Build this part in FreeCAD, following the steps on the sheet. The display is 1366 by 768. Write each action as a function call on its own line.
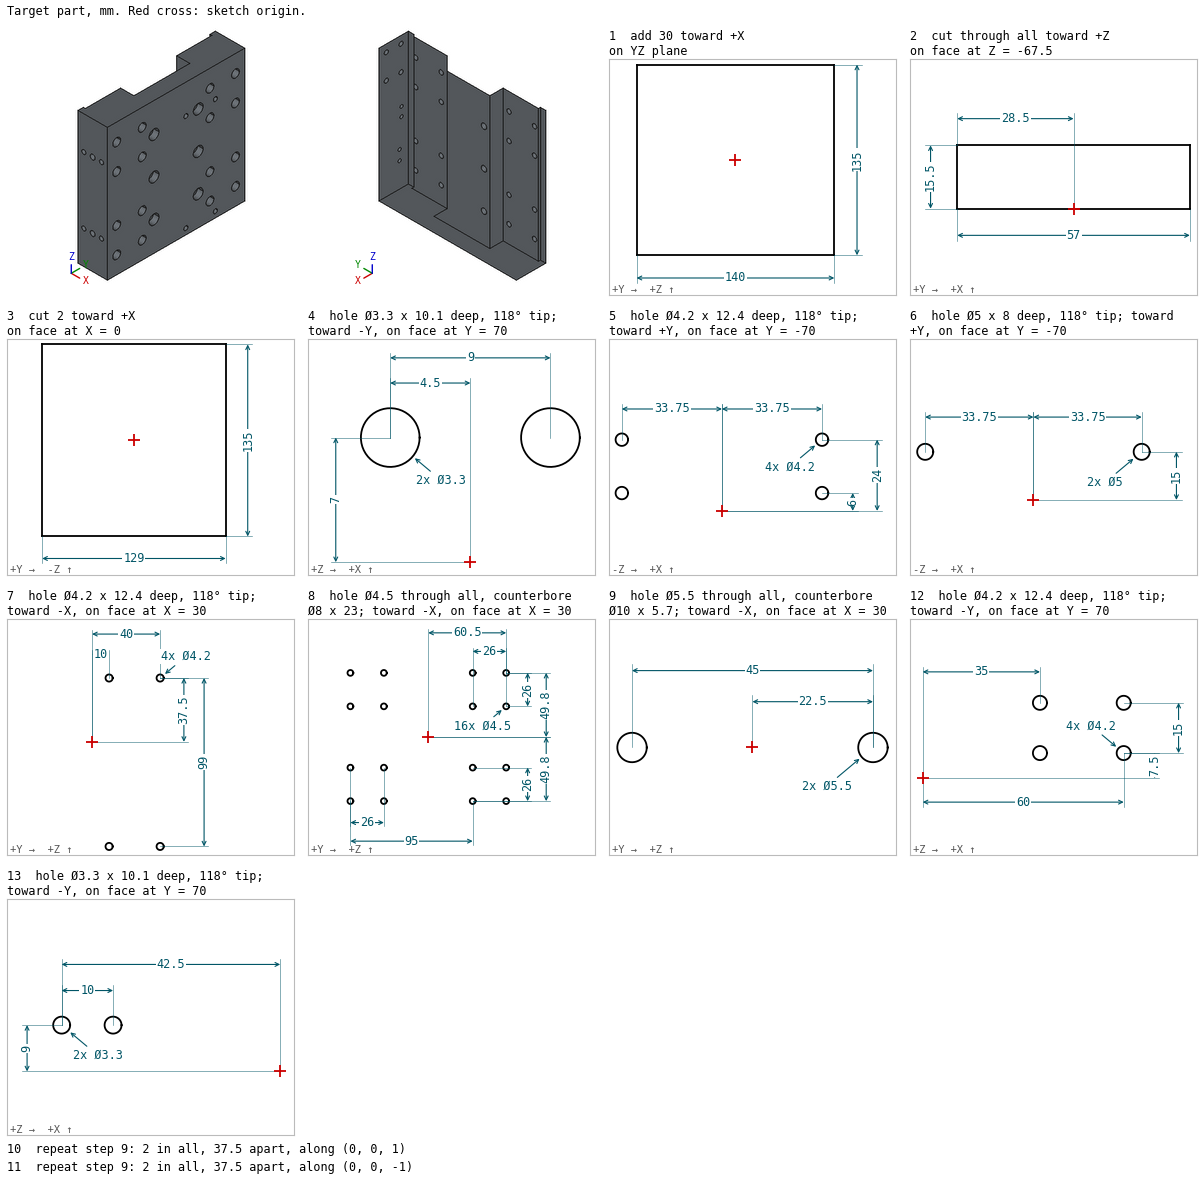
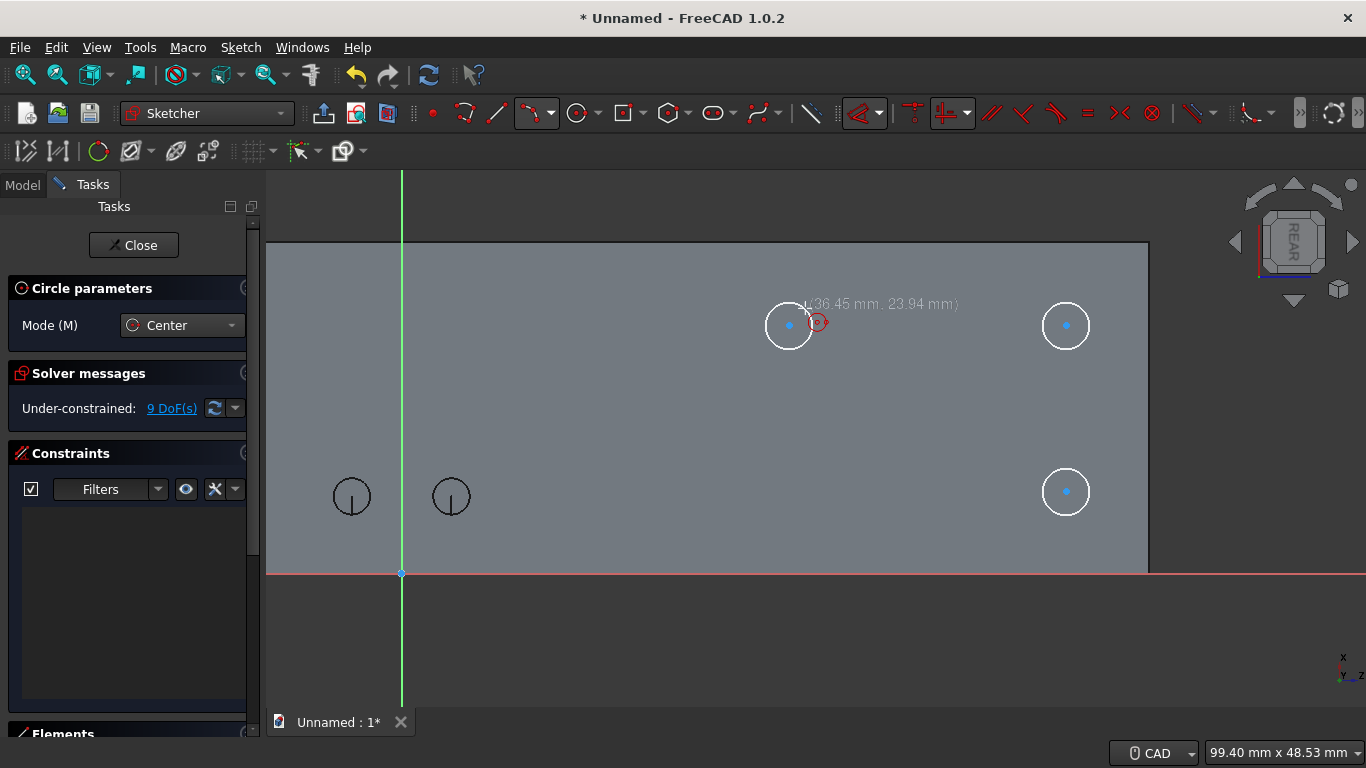
click(789, 491)
click(805, 474)
key(Escape)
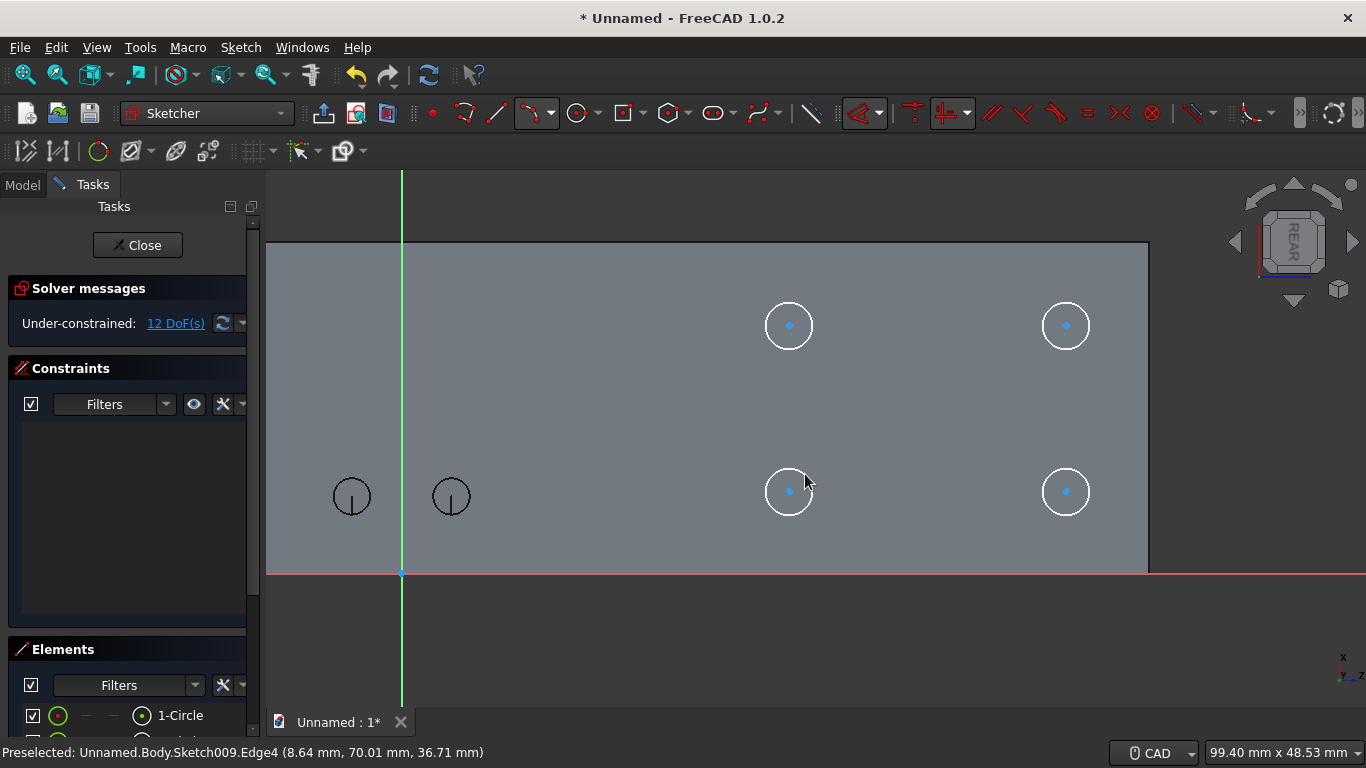
click(1082, 475)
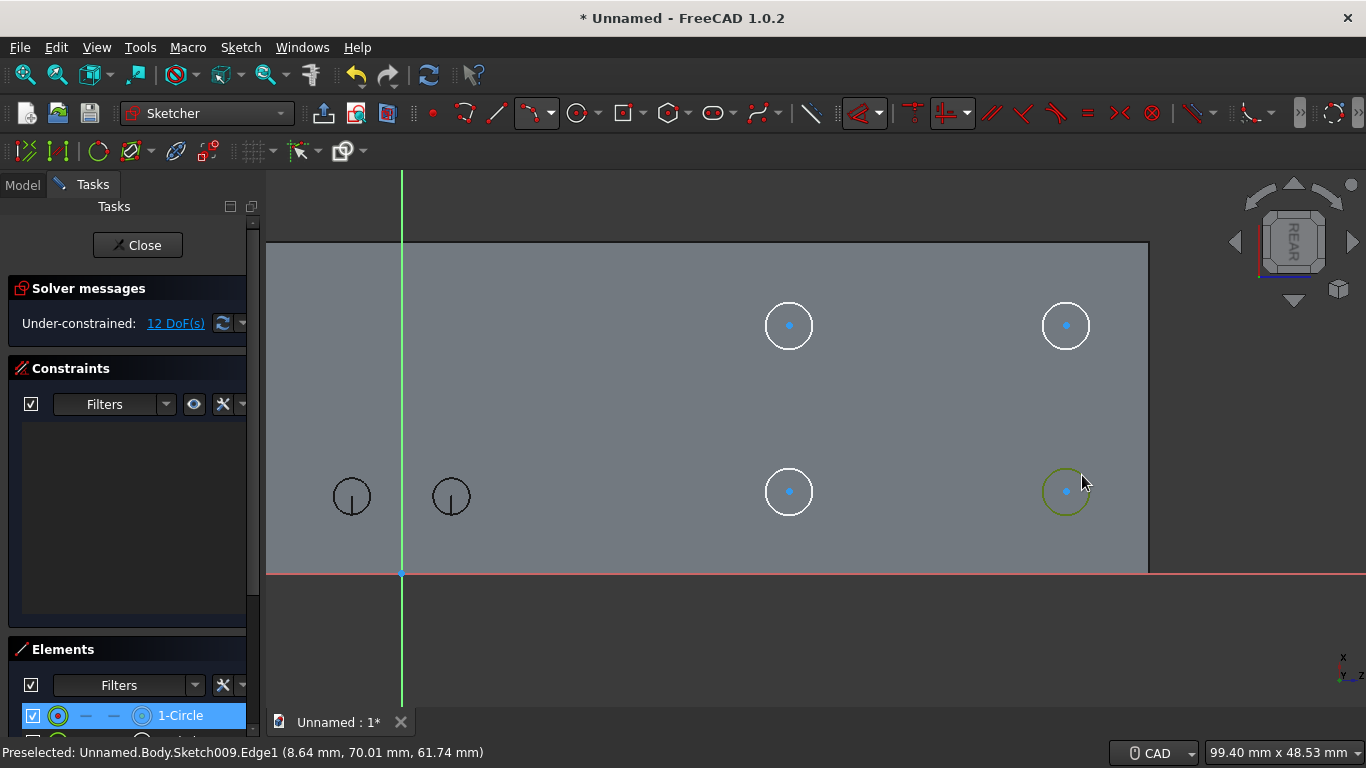
click(1082, 309)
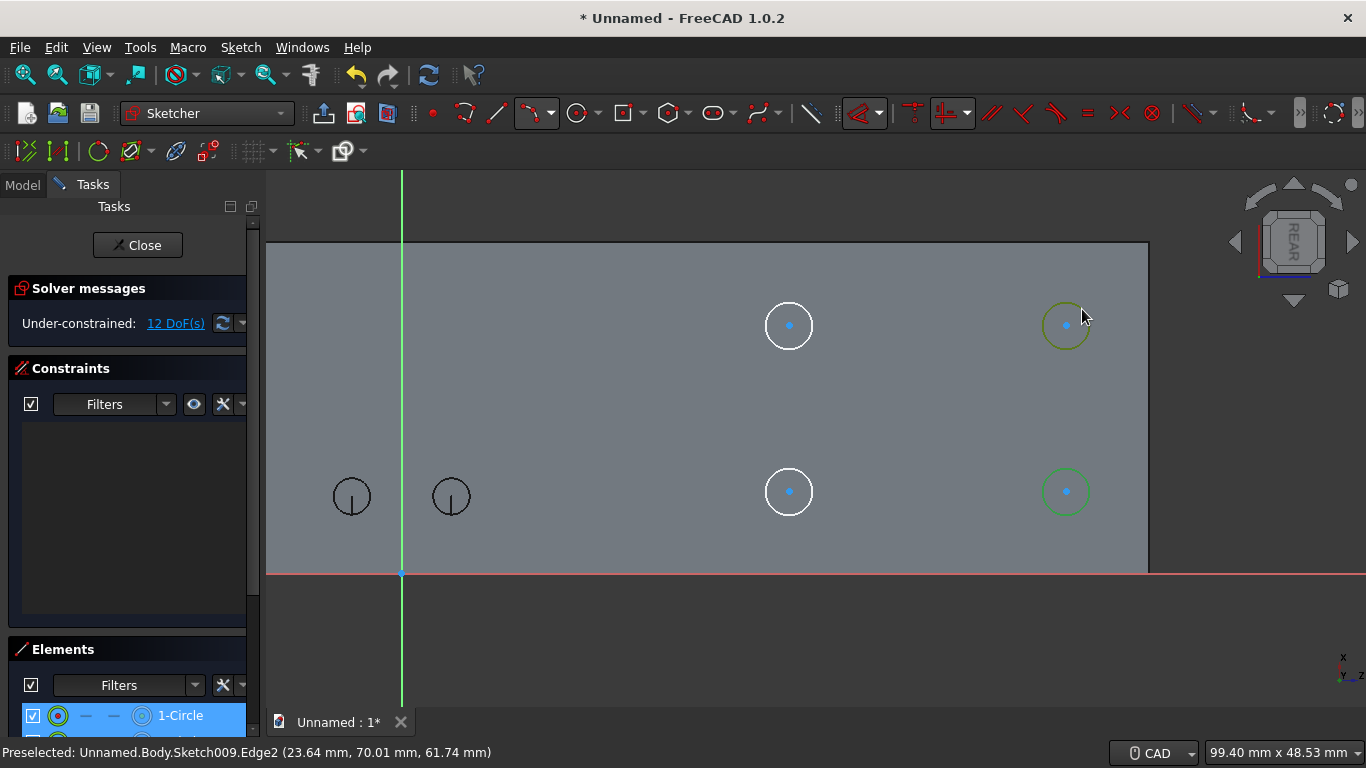
click(805, 309)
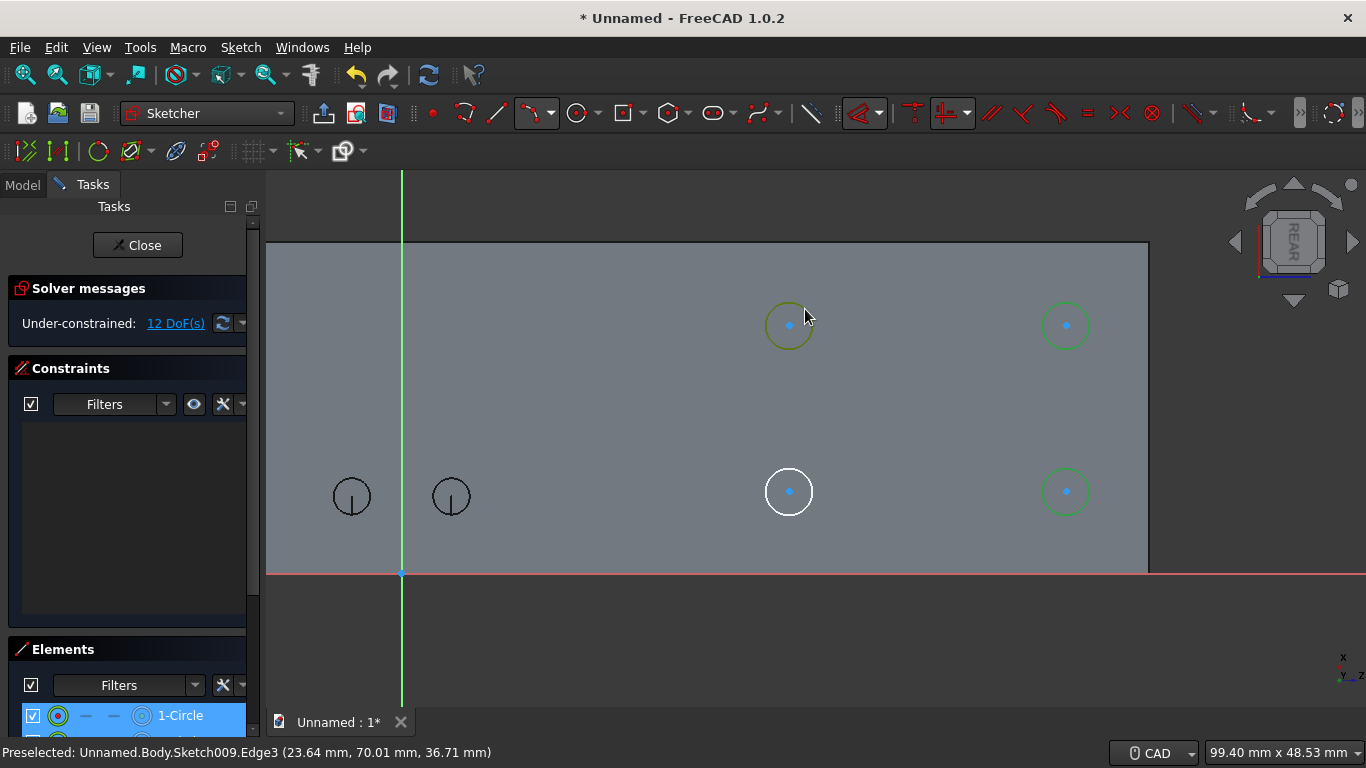
click(805, 475)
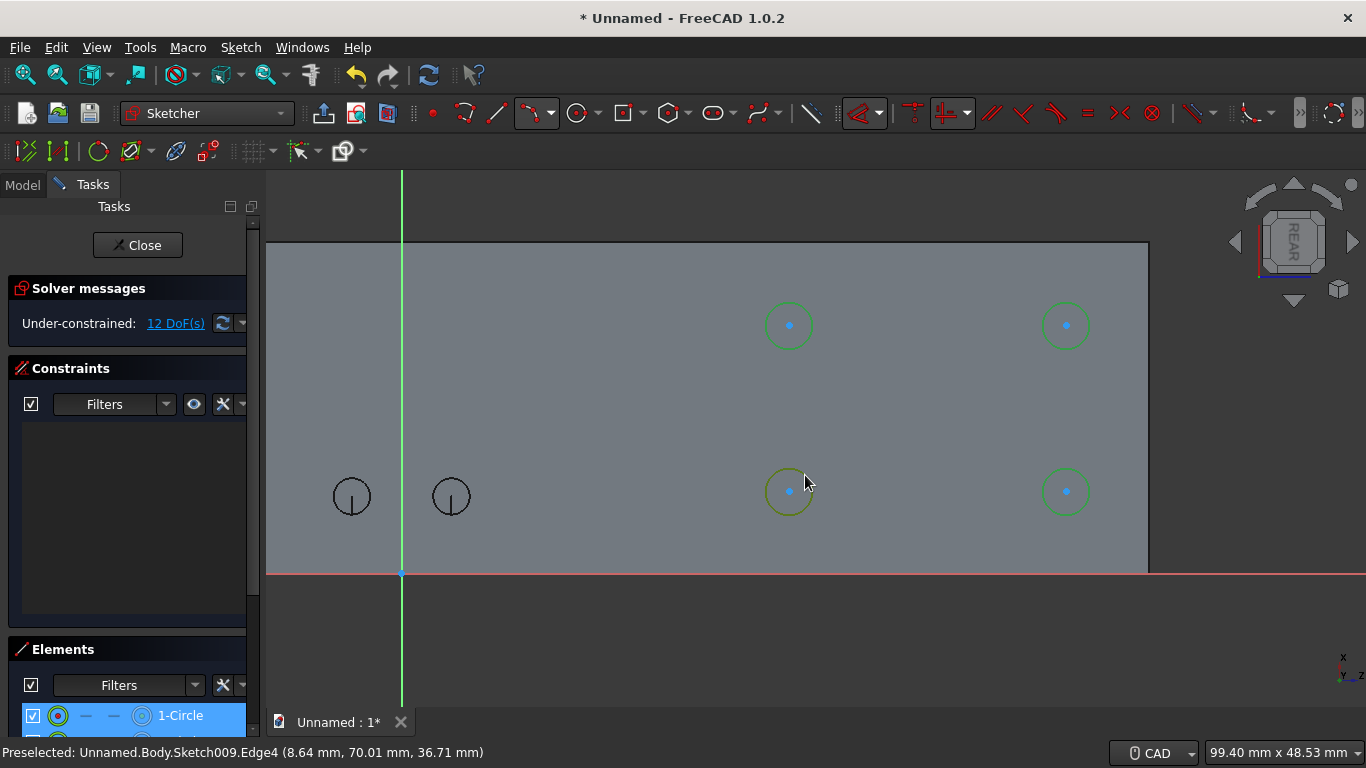
click(1088, 114)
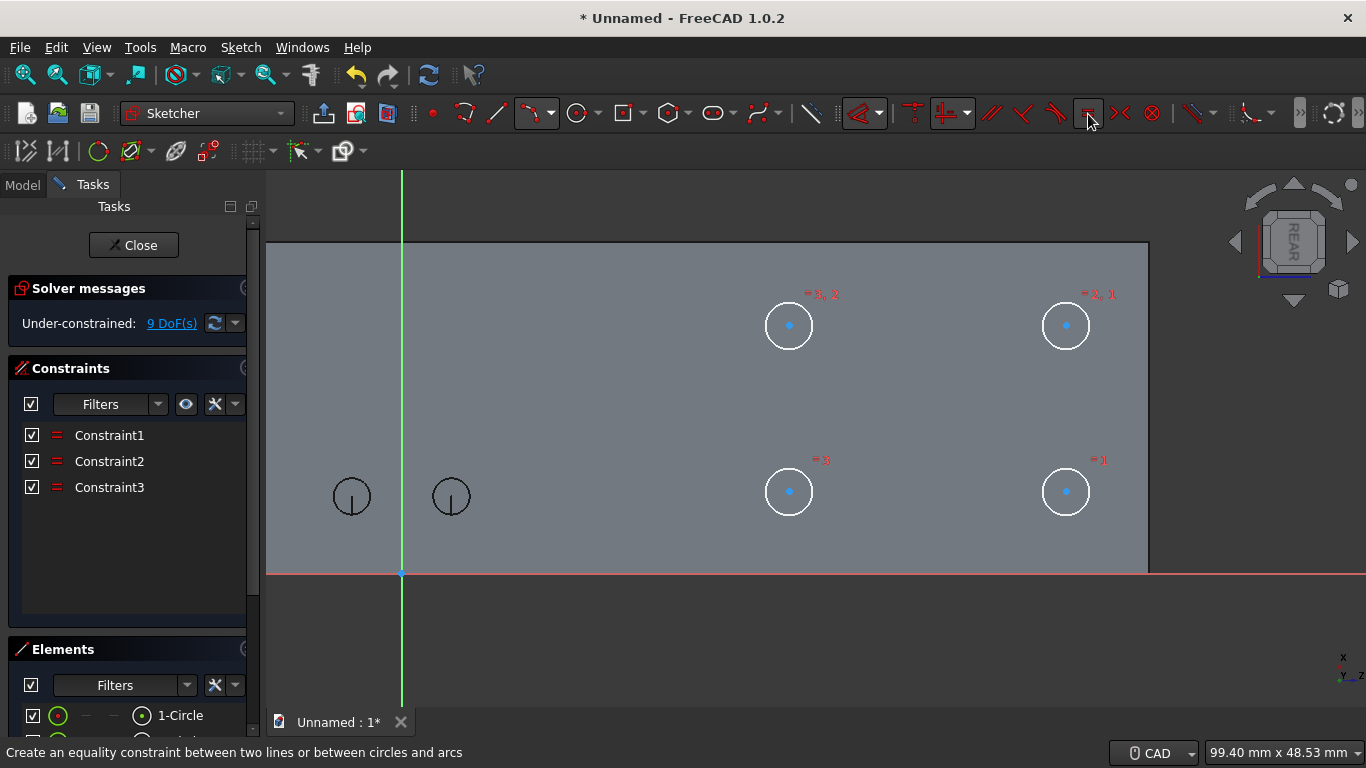
click(1066, 492)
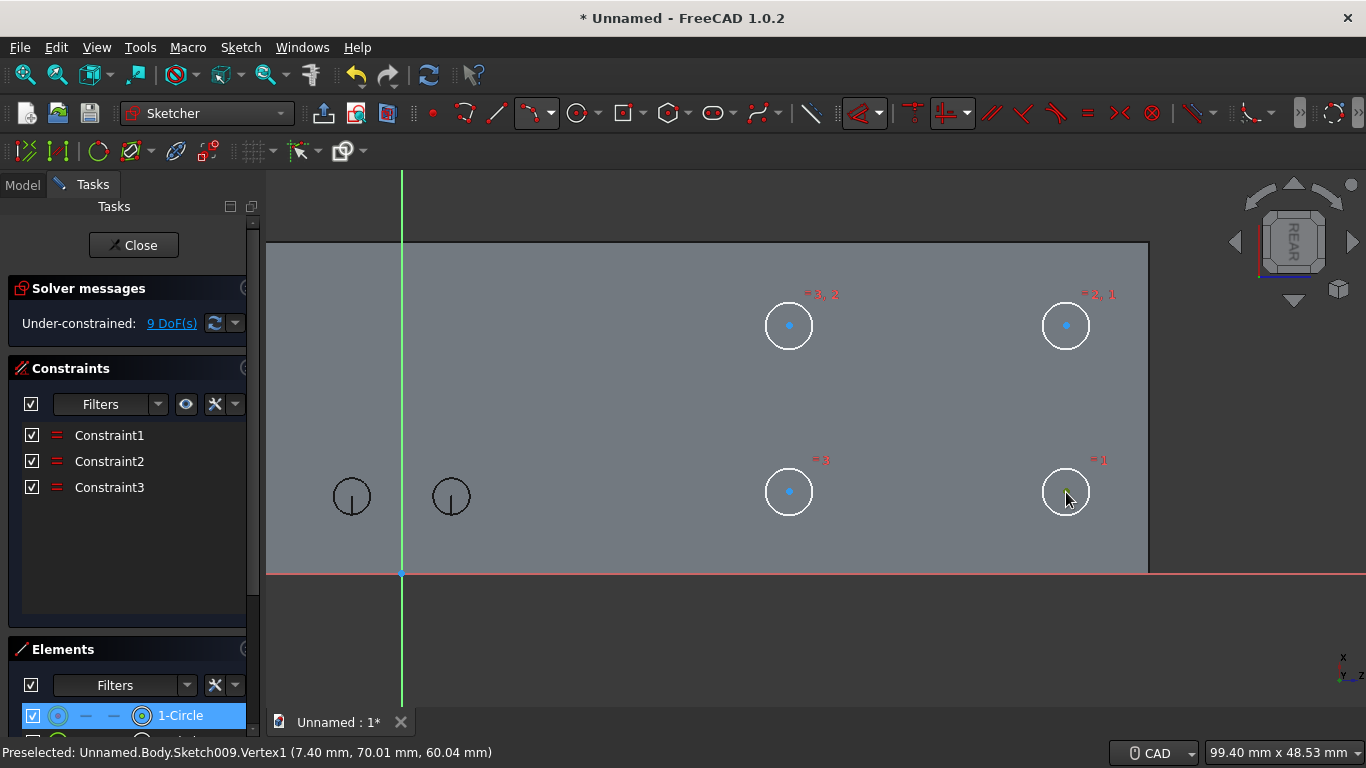
click(1066, 326)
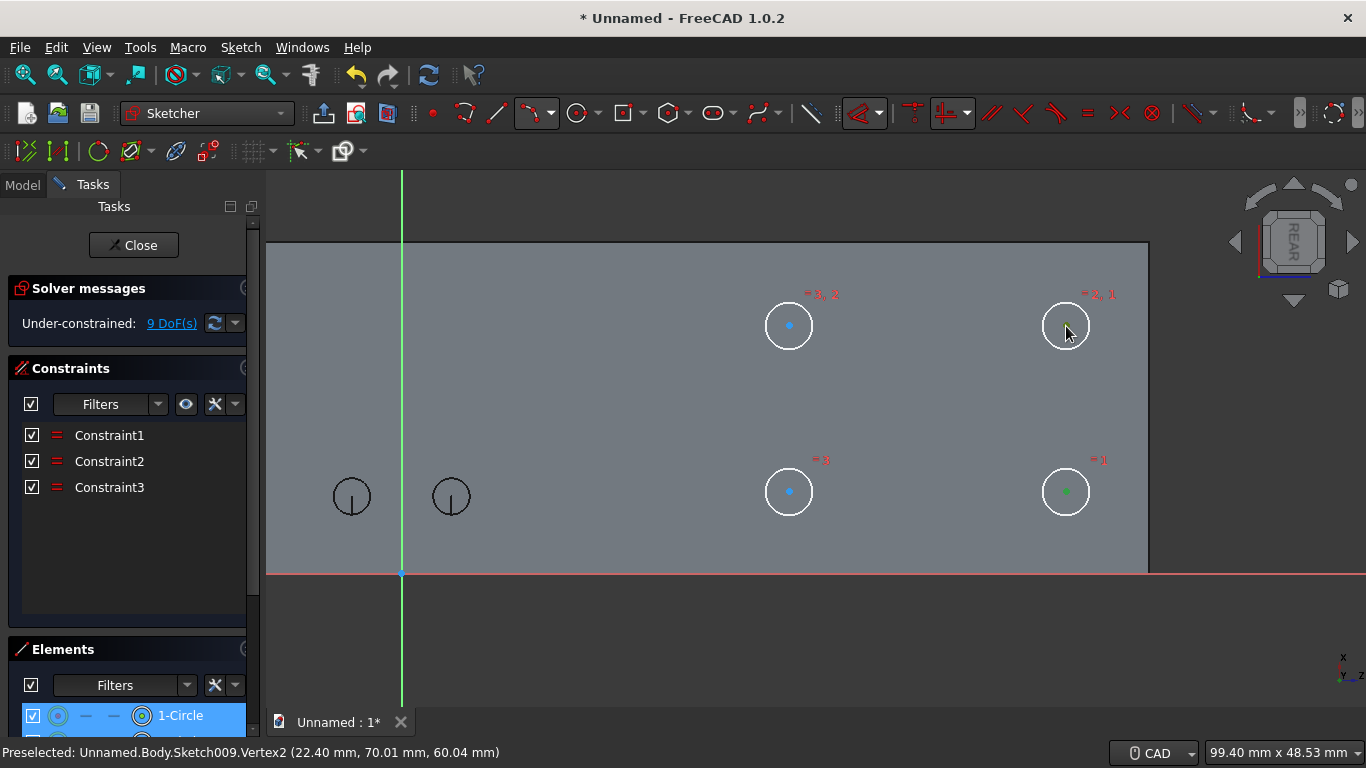
click(970, 114)